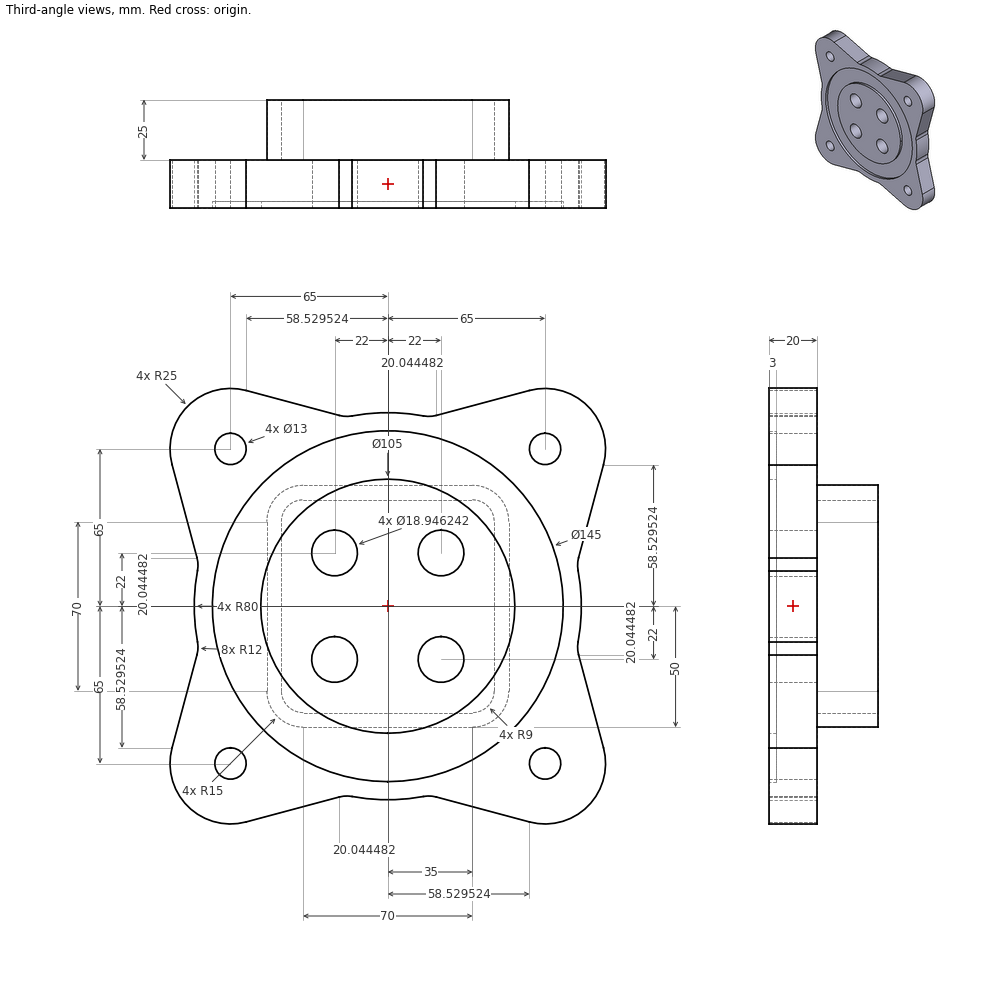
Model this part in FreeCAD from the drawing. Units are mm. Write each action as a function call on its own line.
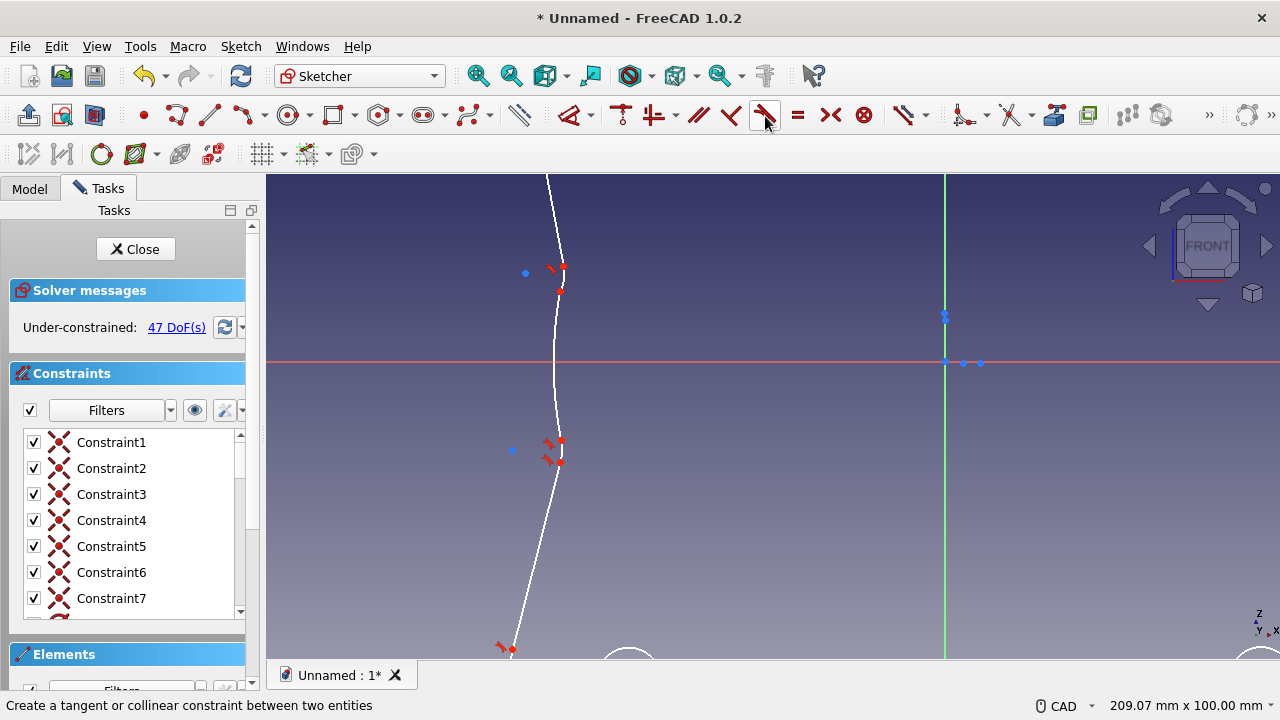
click(555, 336)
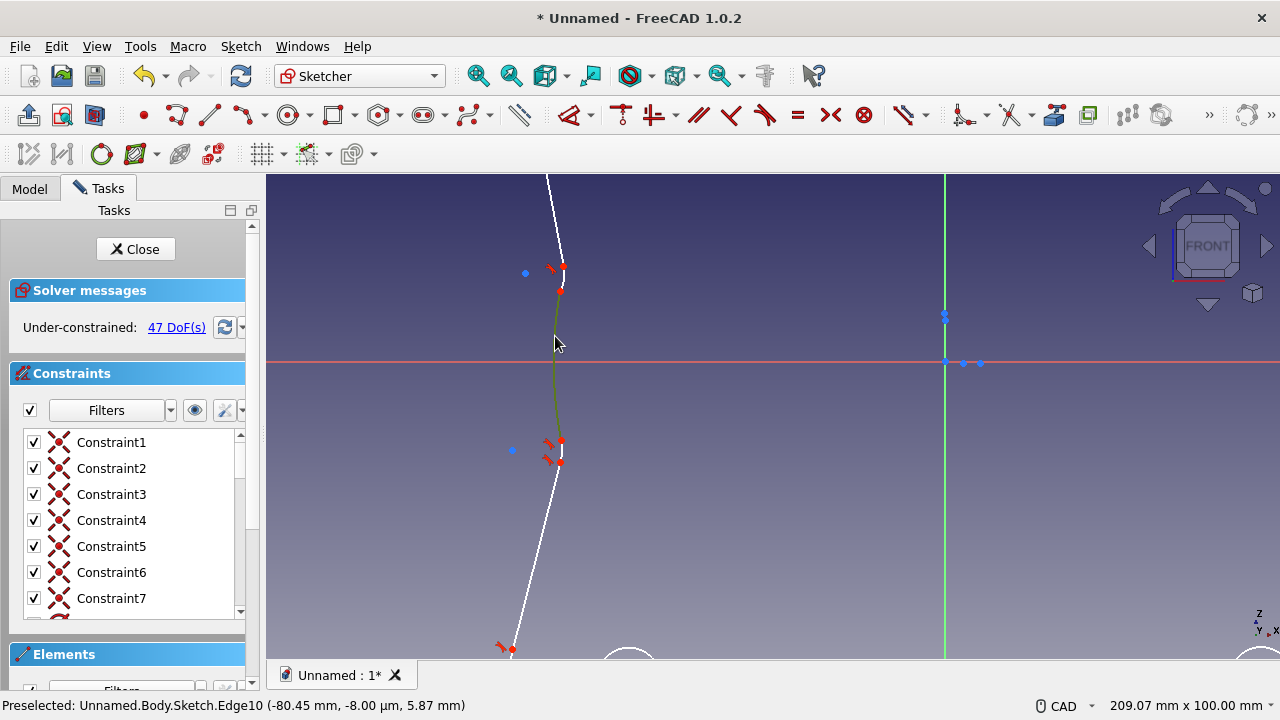
click(564, 279)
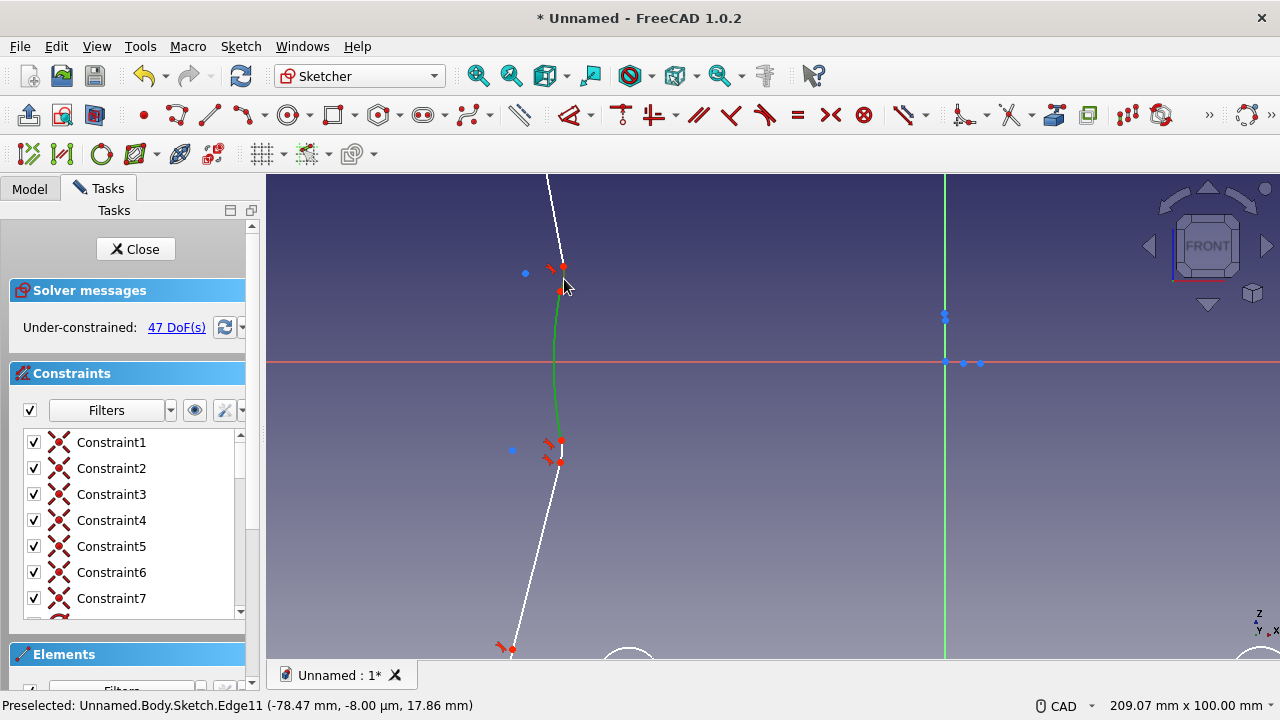
key(t)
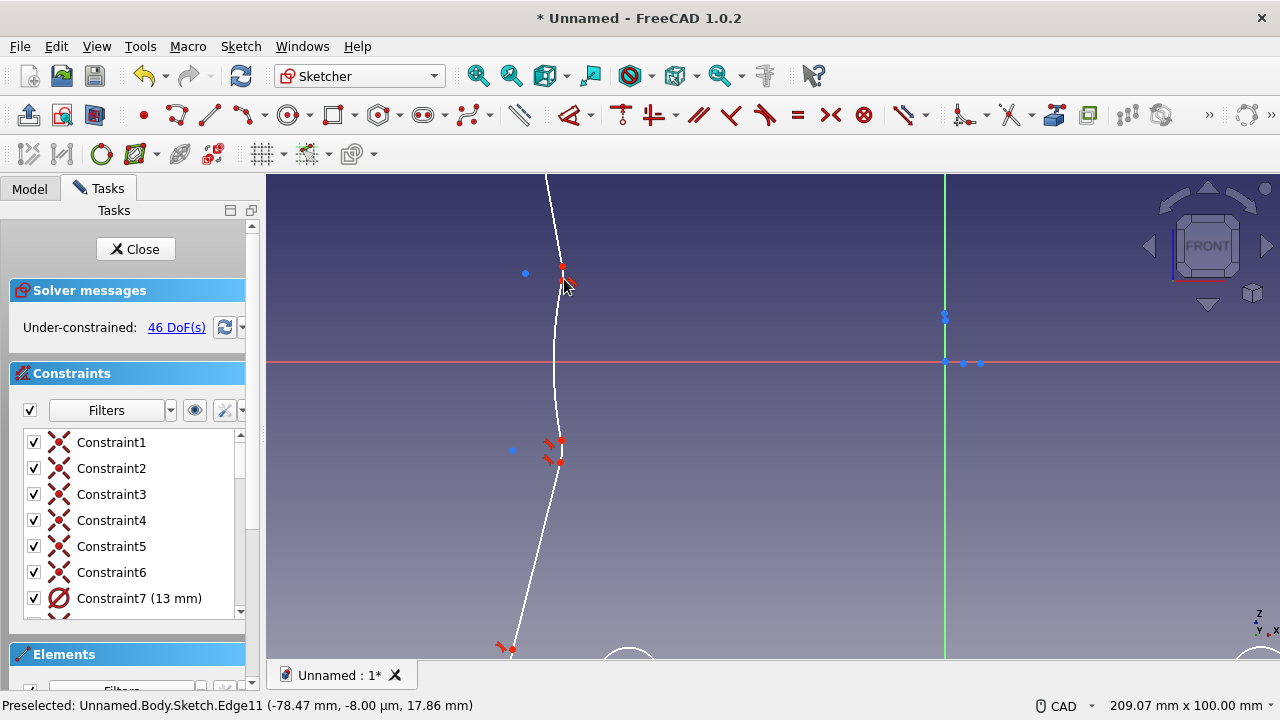
scroll(565, 448, down, 5)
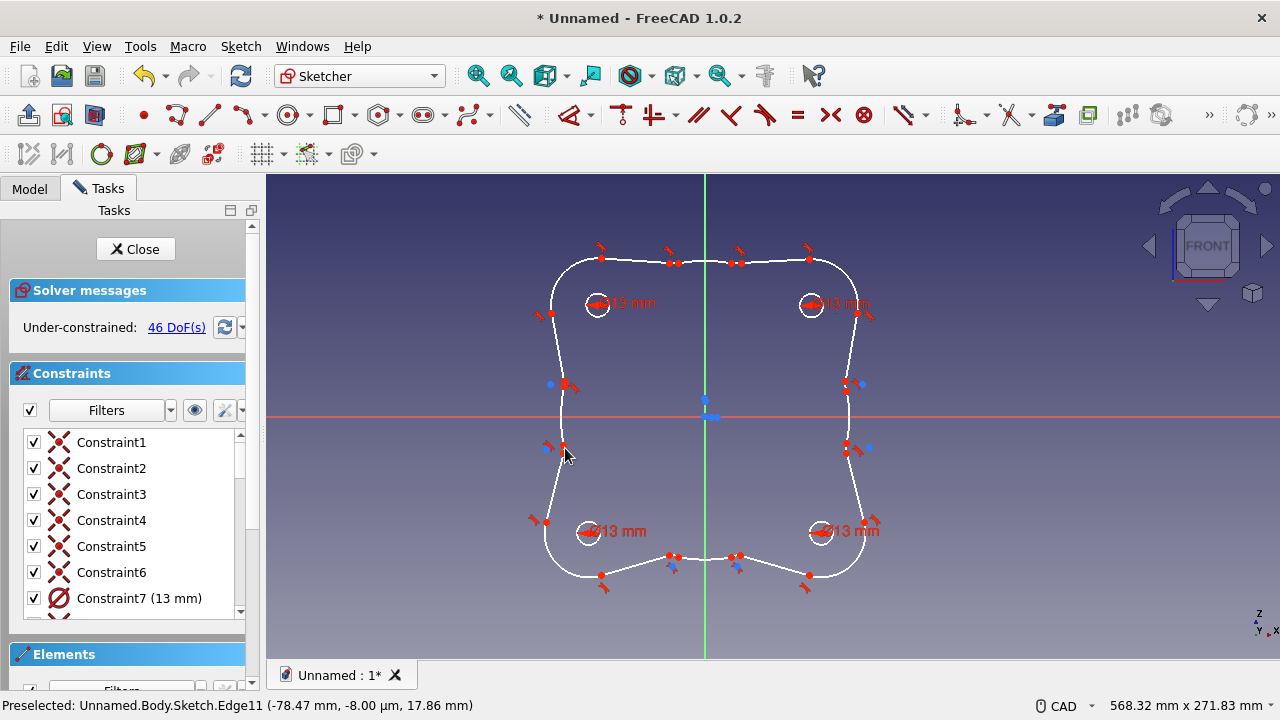
scroll(674, 263, up, 6)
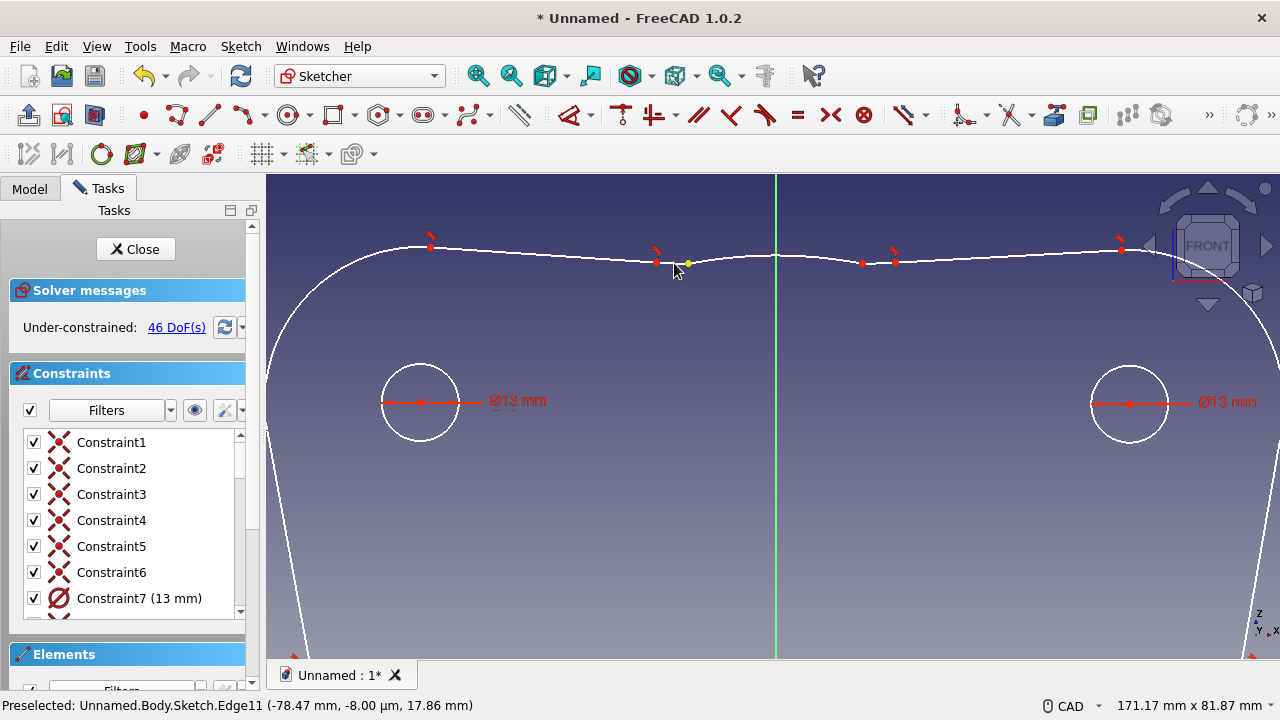
click(673, 263)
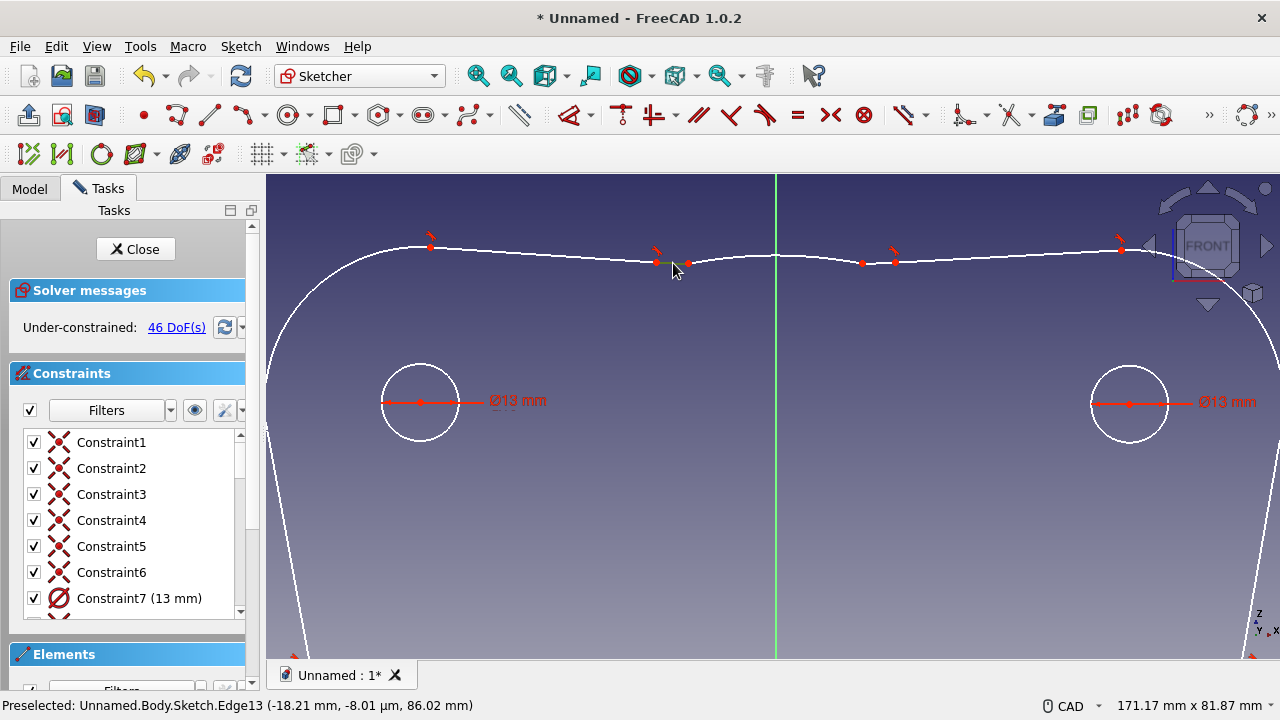
click(811, 257)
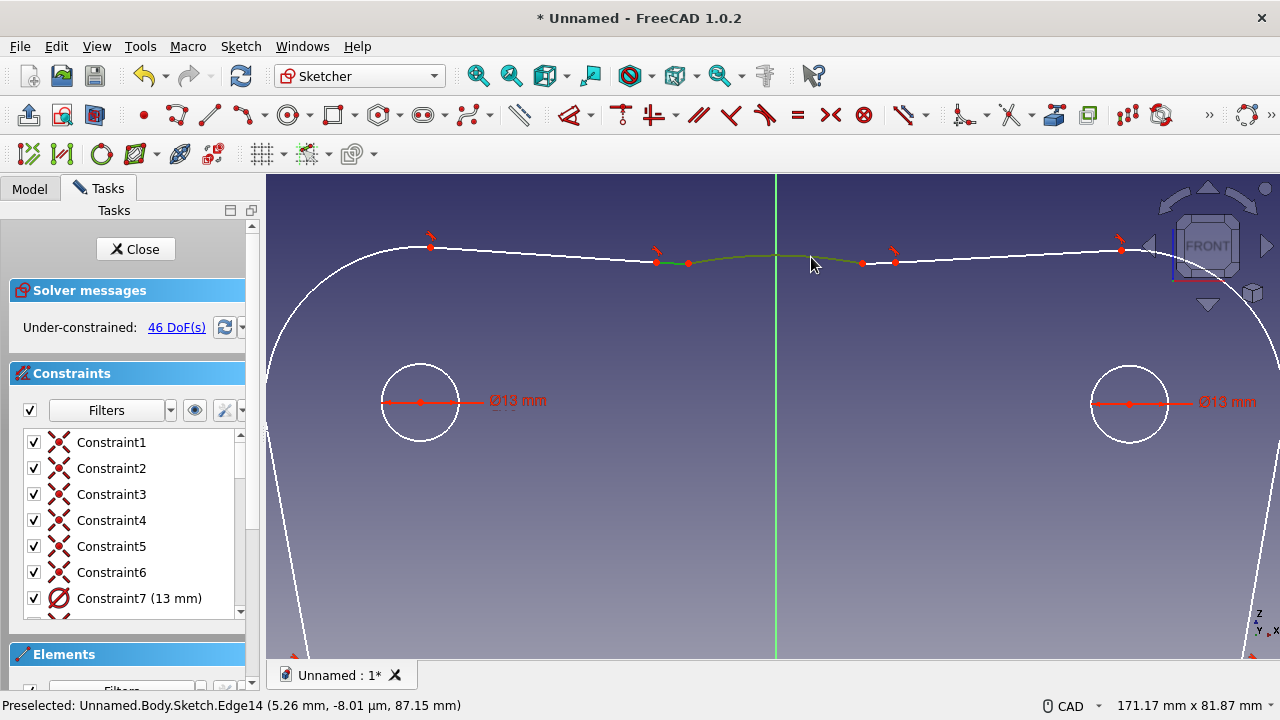
click(765, 116)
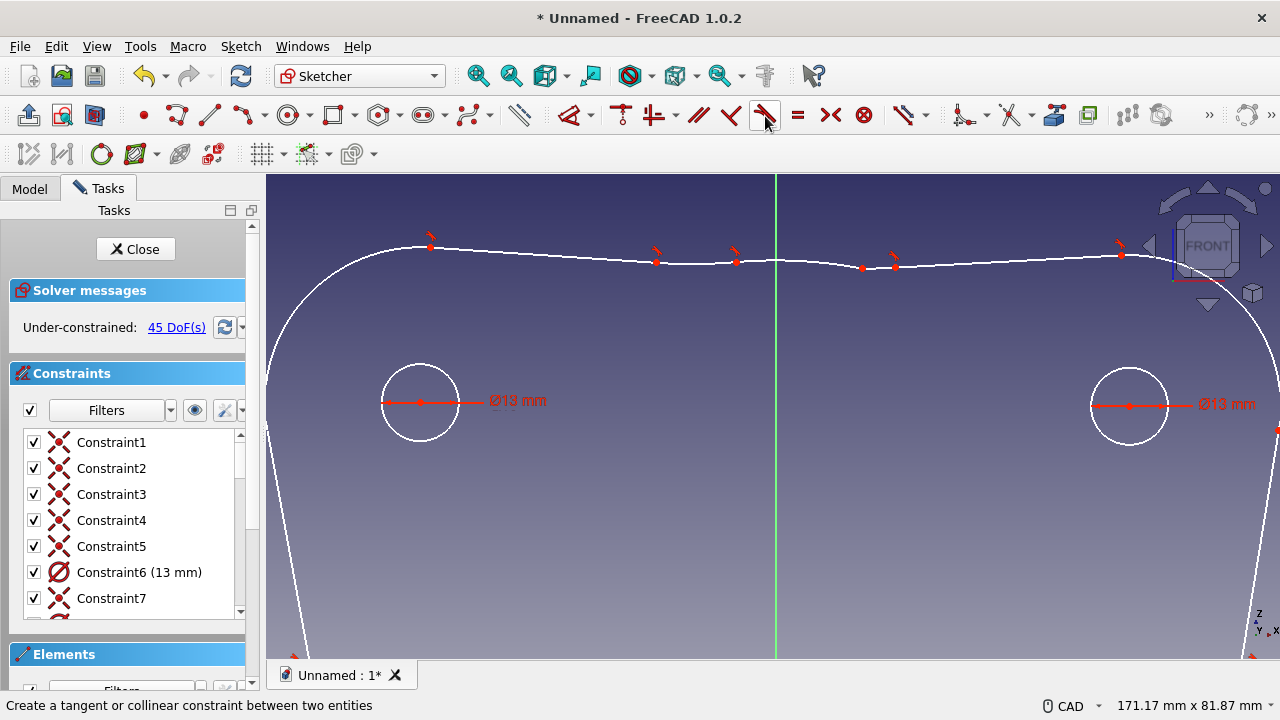
click(825, 263)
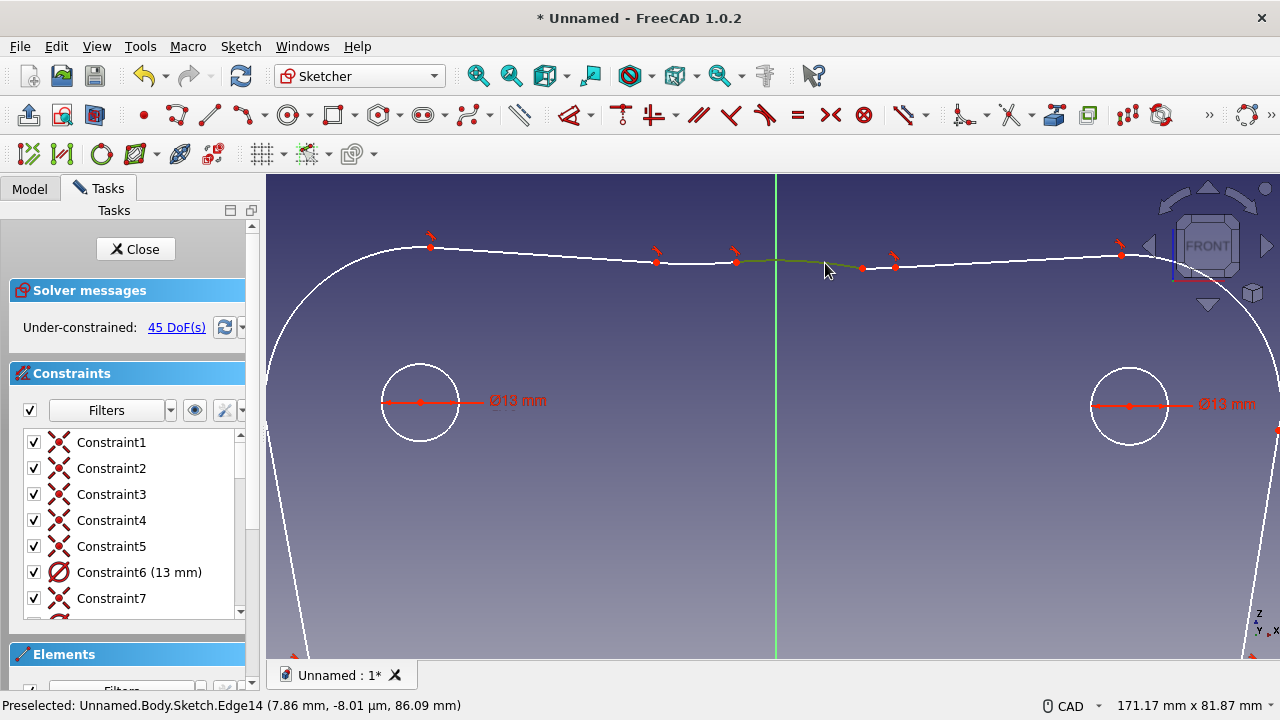
scroll(872, 269, up, 2)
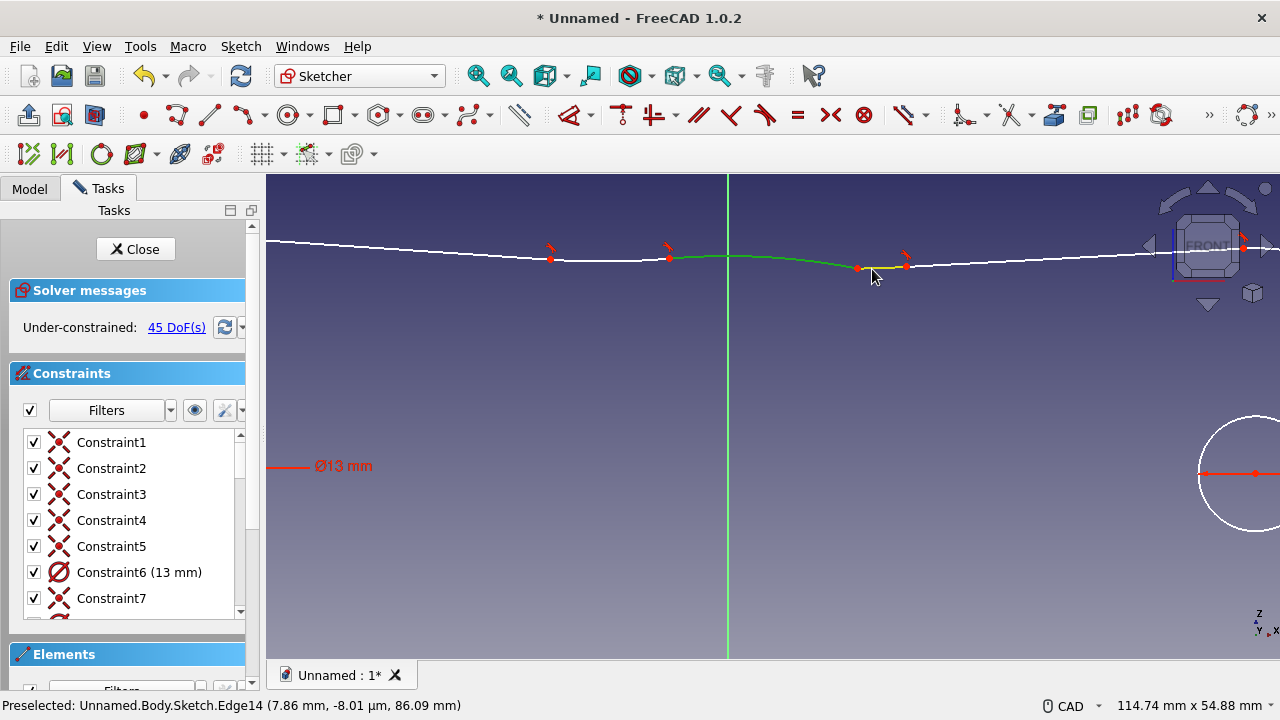
click(872, 268)